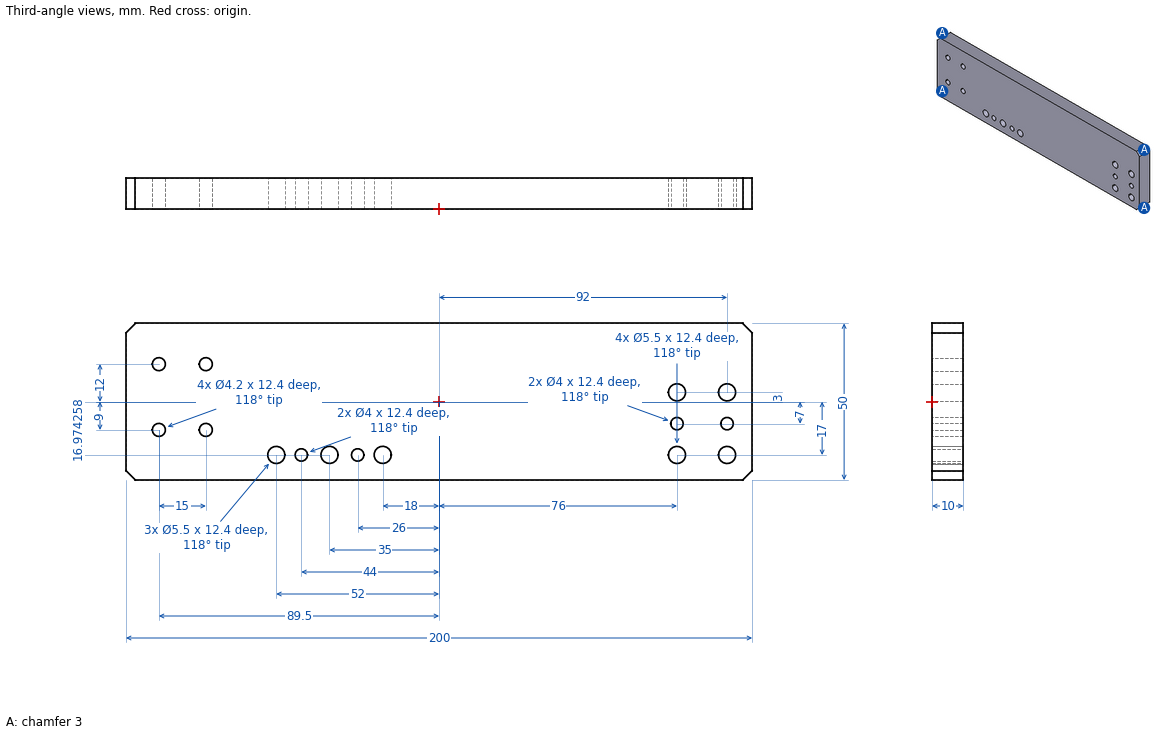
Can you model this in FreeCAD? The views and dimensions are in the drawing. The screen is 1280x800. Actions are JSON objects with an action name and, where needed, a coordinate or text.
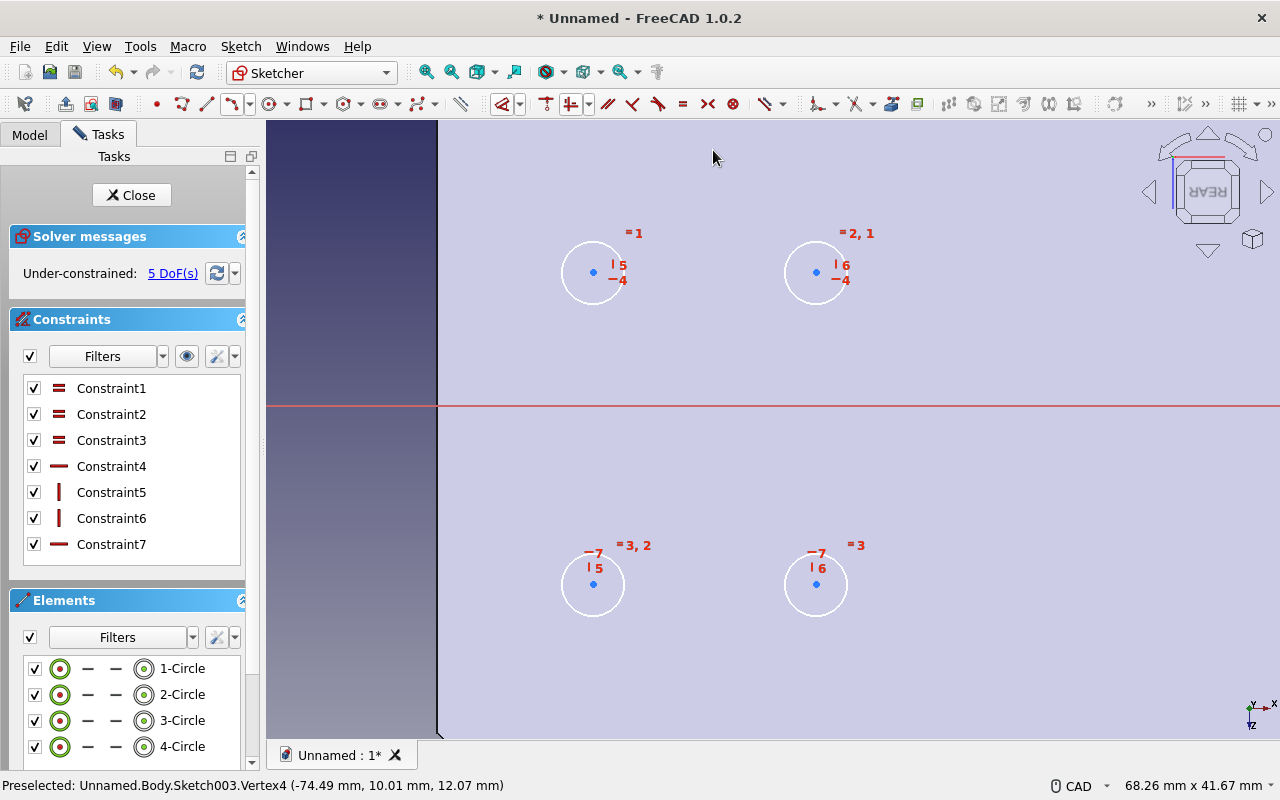
{"action": "left_click", "coordinate": [502, 104]}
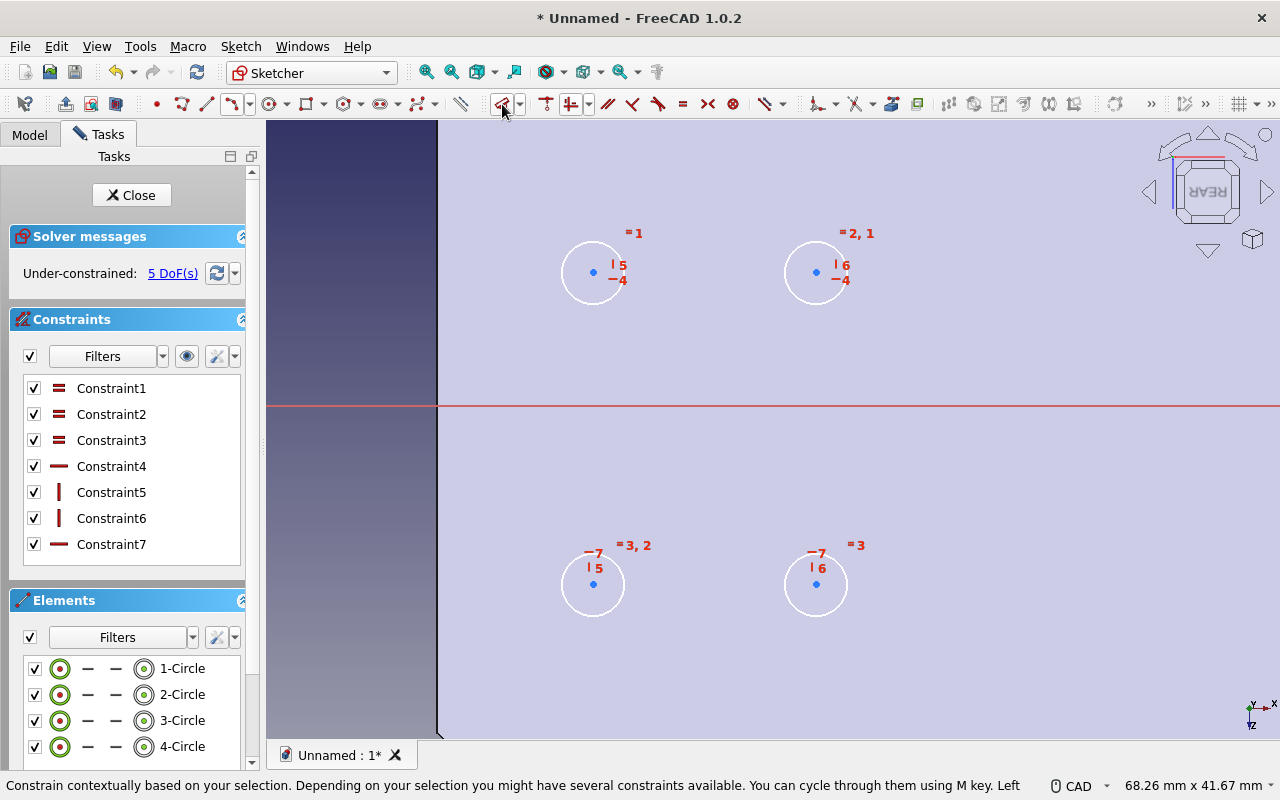
{"action": "left_click", "coordinate": [615, 251]}
{"action": "left_click", "coordinate": [638, 228]}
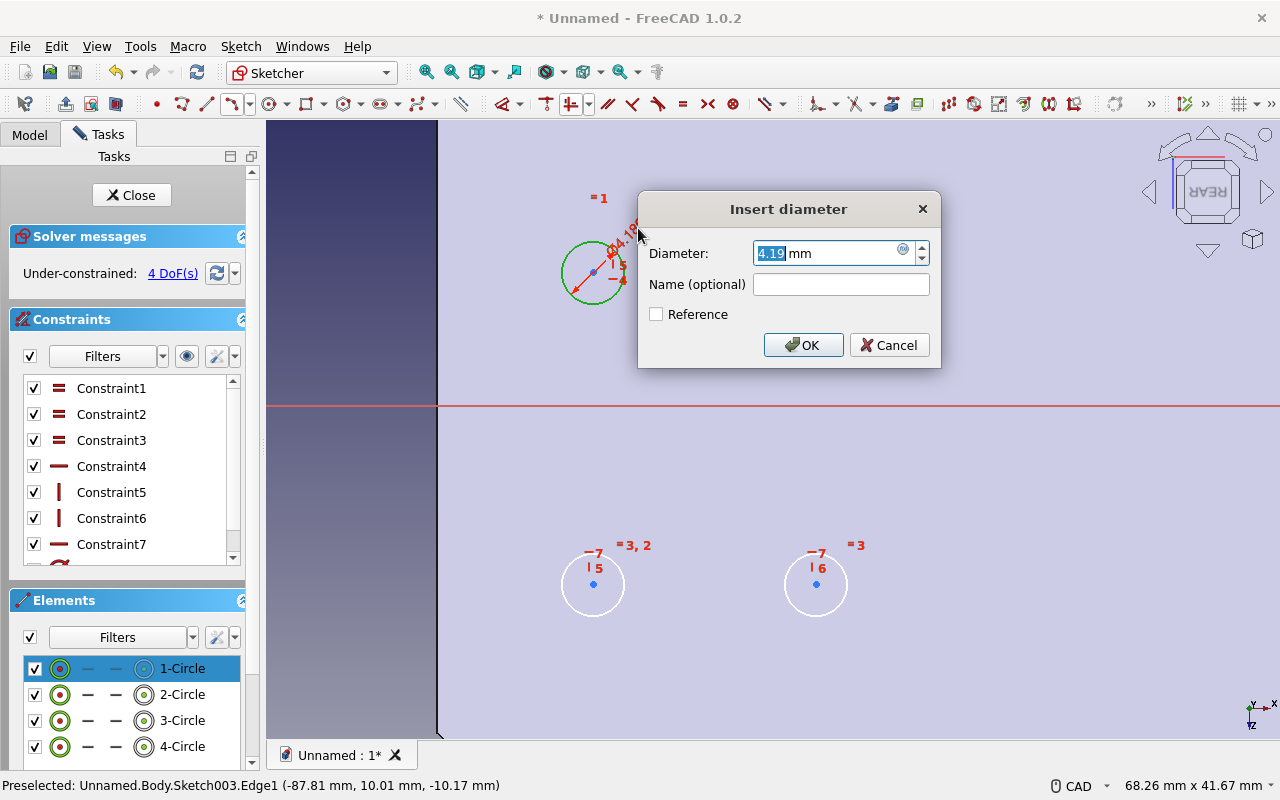
{"action": "type", "text": "4.2"}
{"action": "key", "text": "Return"}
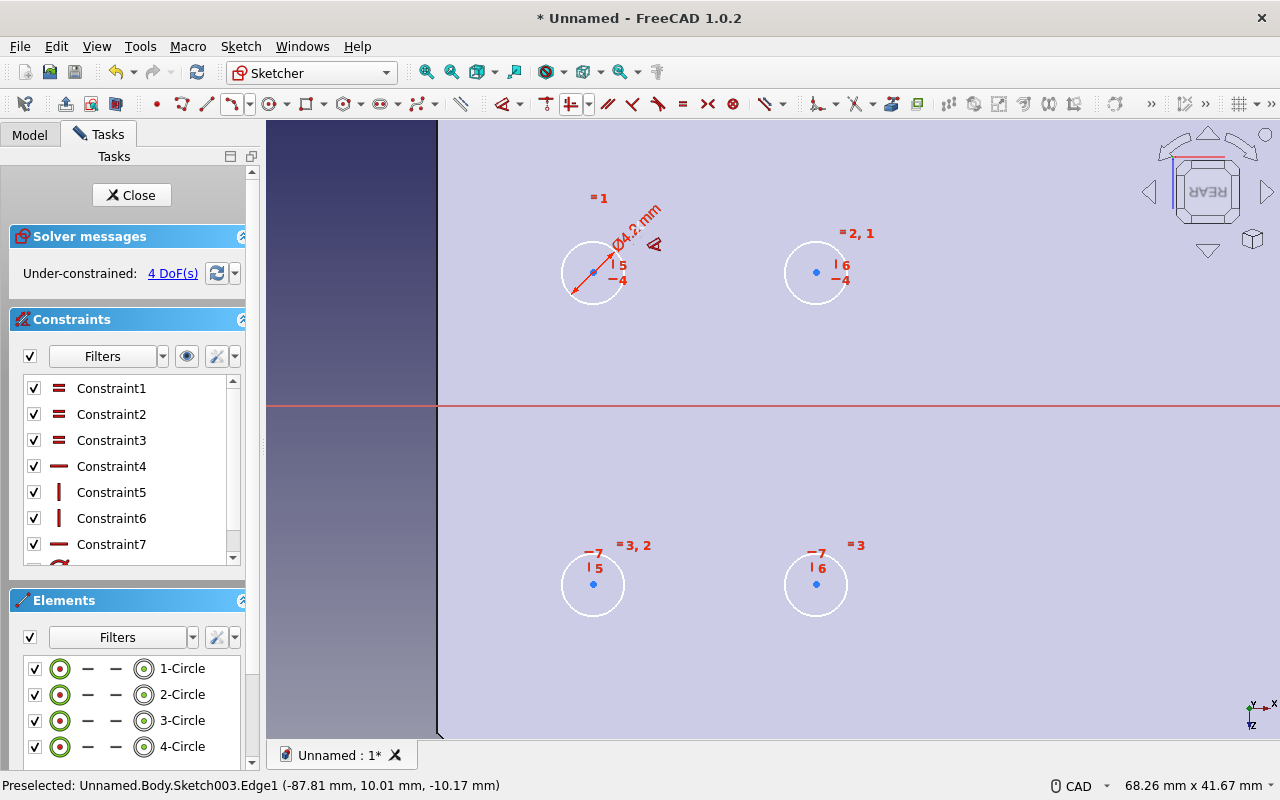
{"action": "left_click", "coordinate": [593, 273]}
{"action": "left_click", "coordinate": [559, 339]}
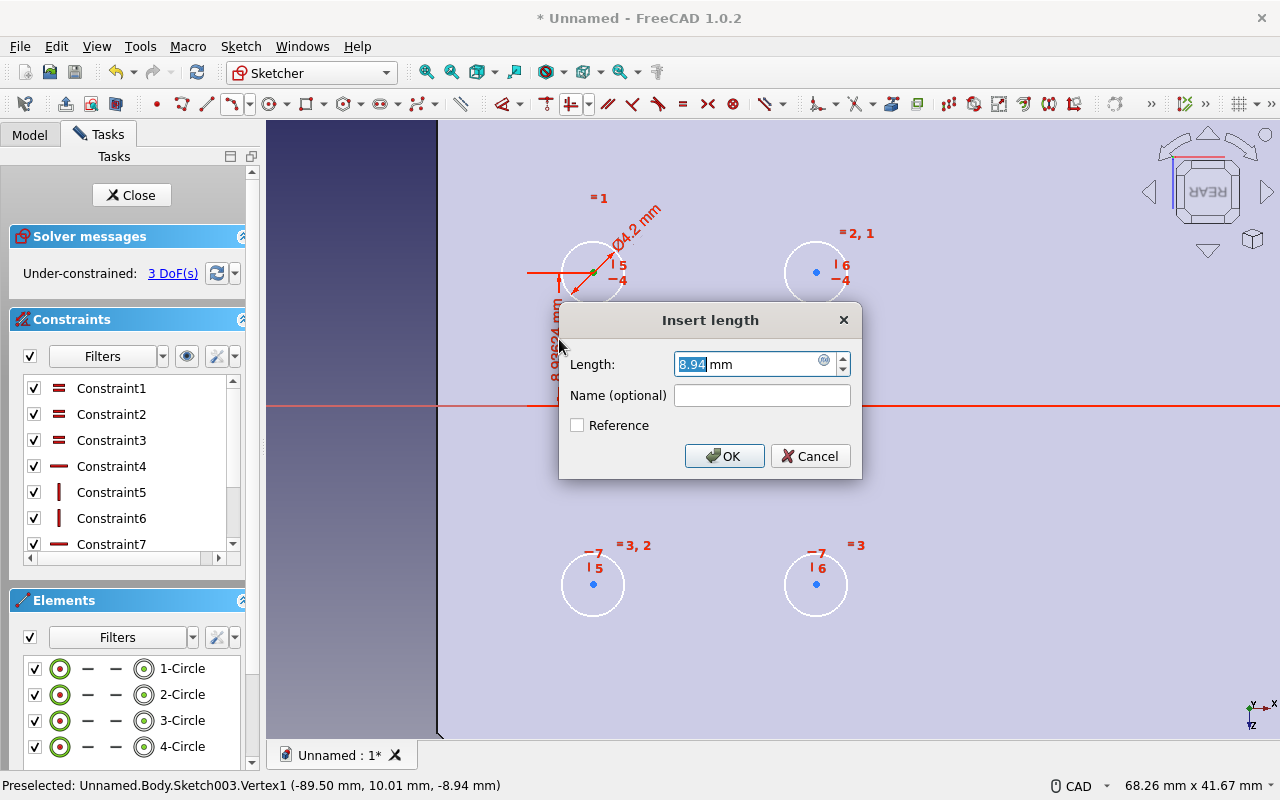
{"action": "type", "text": "9"}
{"action": "key", "text": "Return"}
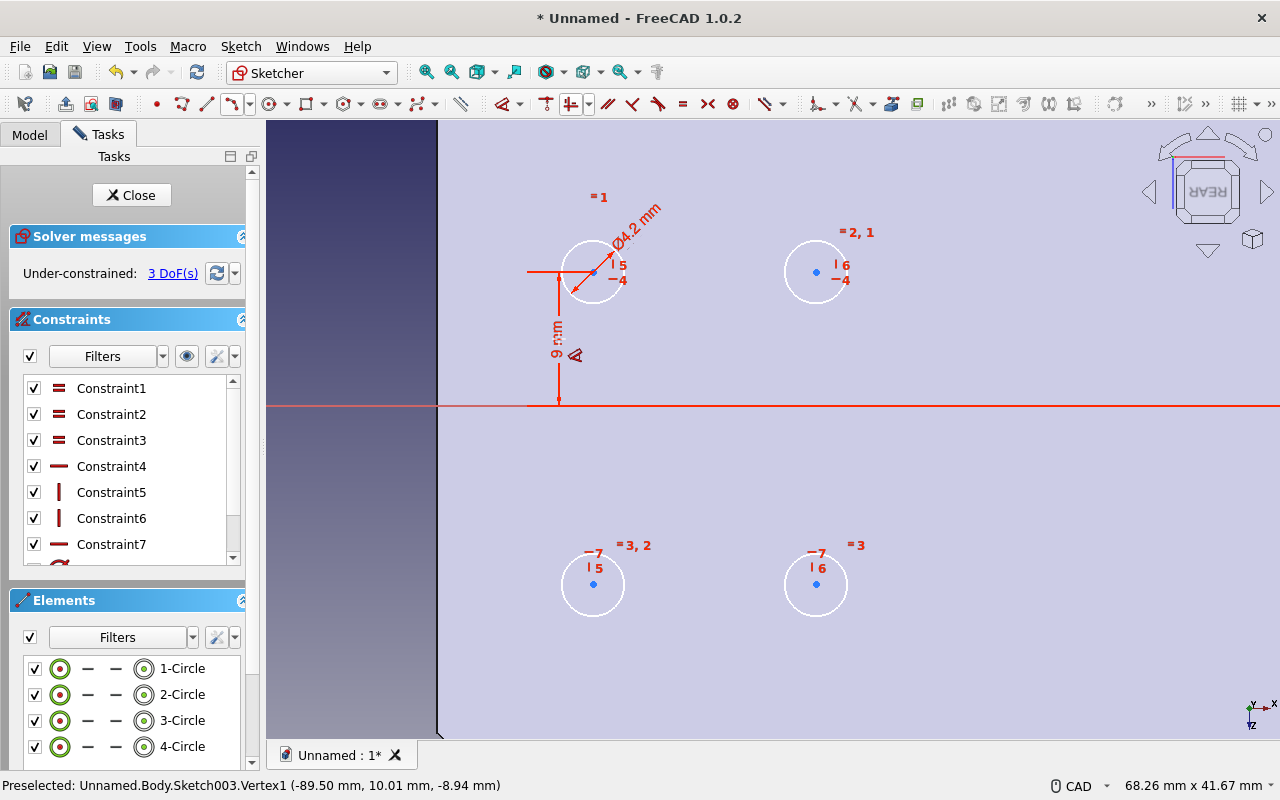
{"action": "left_click", "coordinate": [593, 585]}
{"action": "left_click", "coordinate": [559, 495]}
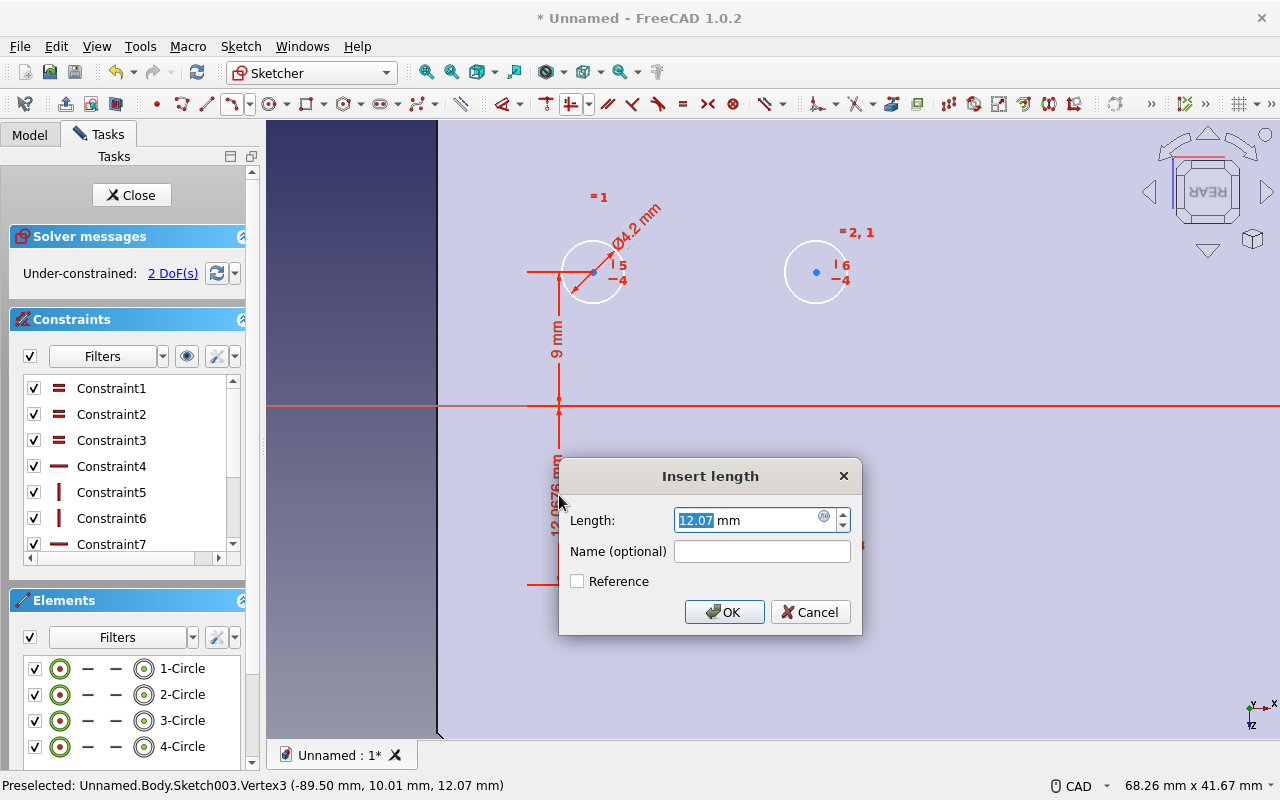
{"action": "type", "text": "12"}
{"action": "key", "text": "Return"}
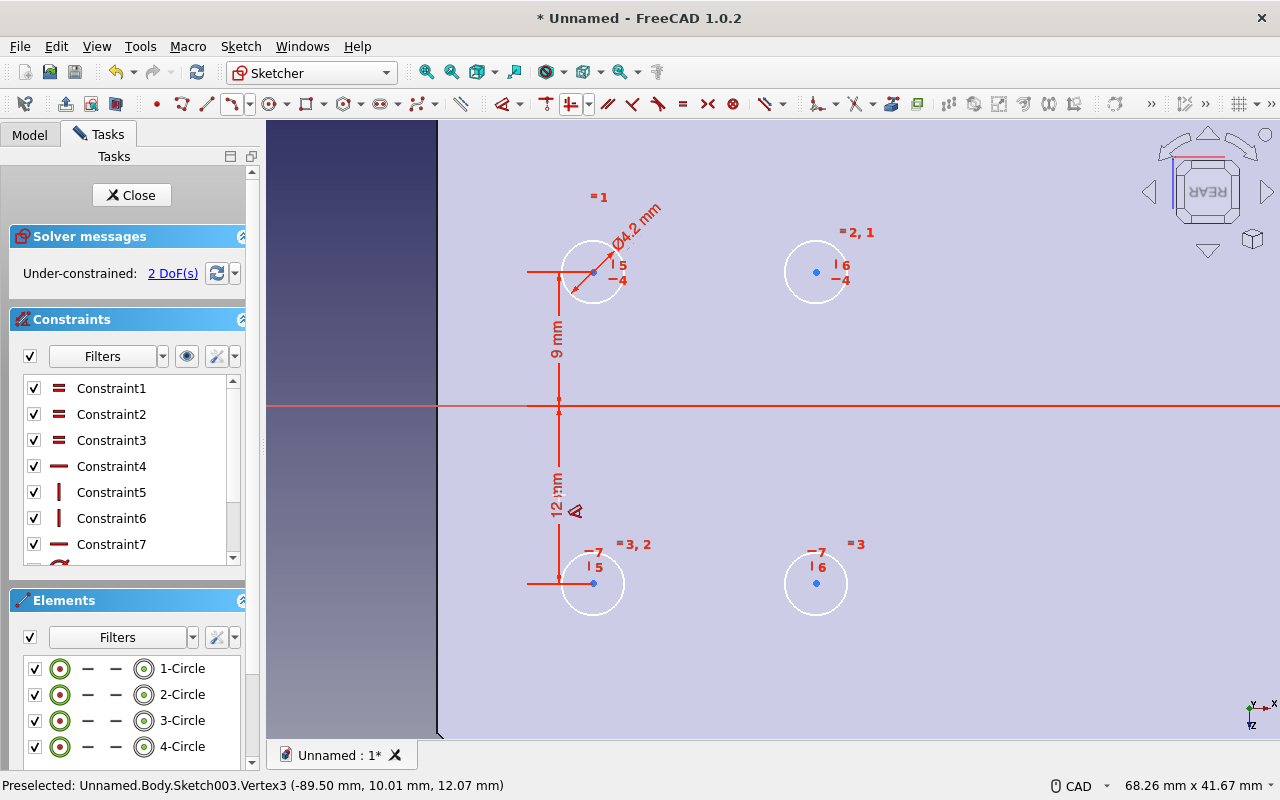
{"action": "left_click", "coordinate": [593, 272]}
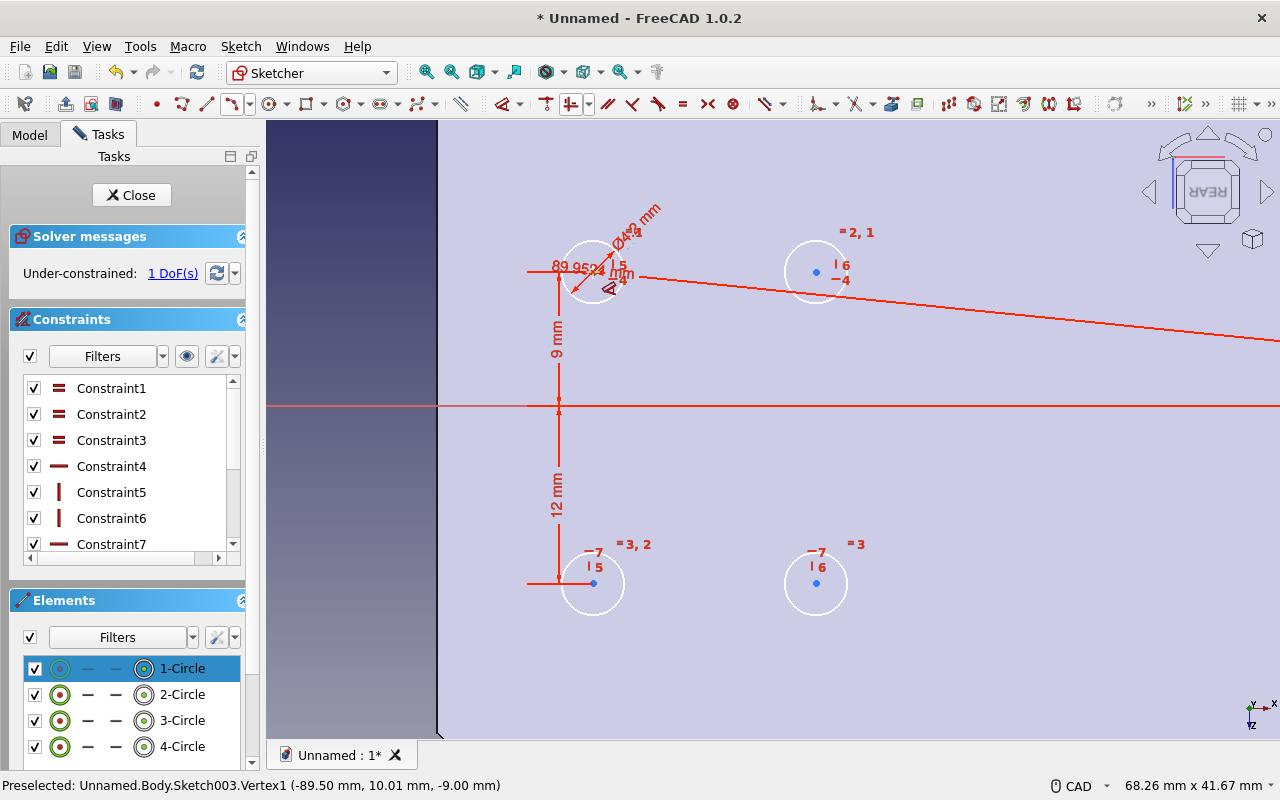
{"action": "left_click", "coordinate": [816, 272]}
{"action": "left_click", "coordinate": [756, 238]}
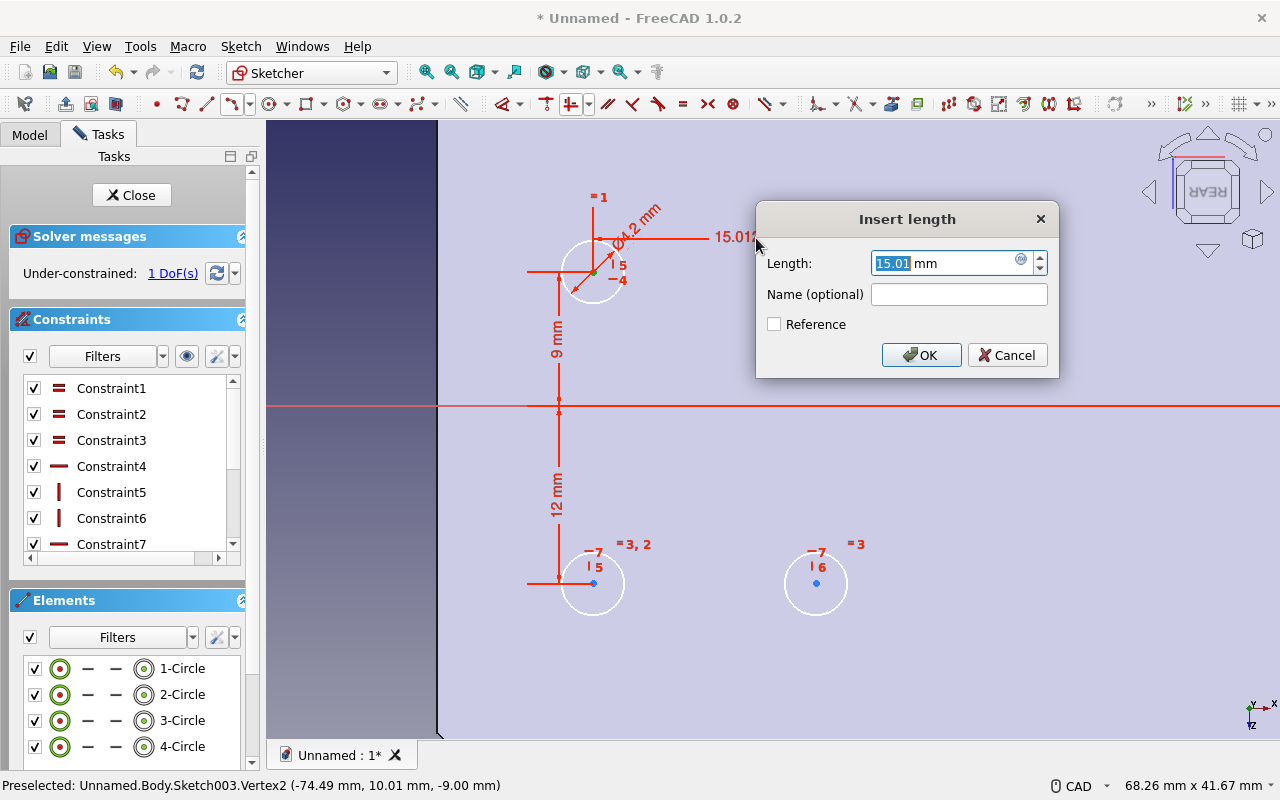
{"action": "type", "text": "15"}
{"action": "key", "text": "Return"}